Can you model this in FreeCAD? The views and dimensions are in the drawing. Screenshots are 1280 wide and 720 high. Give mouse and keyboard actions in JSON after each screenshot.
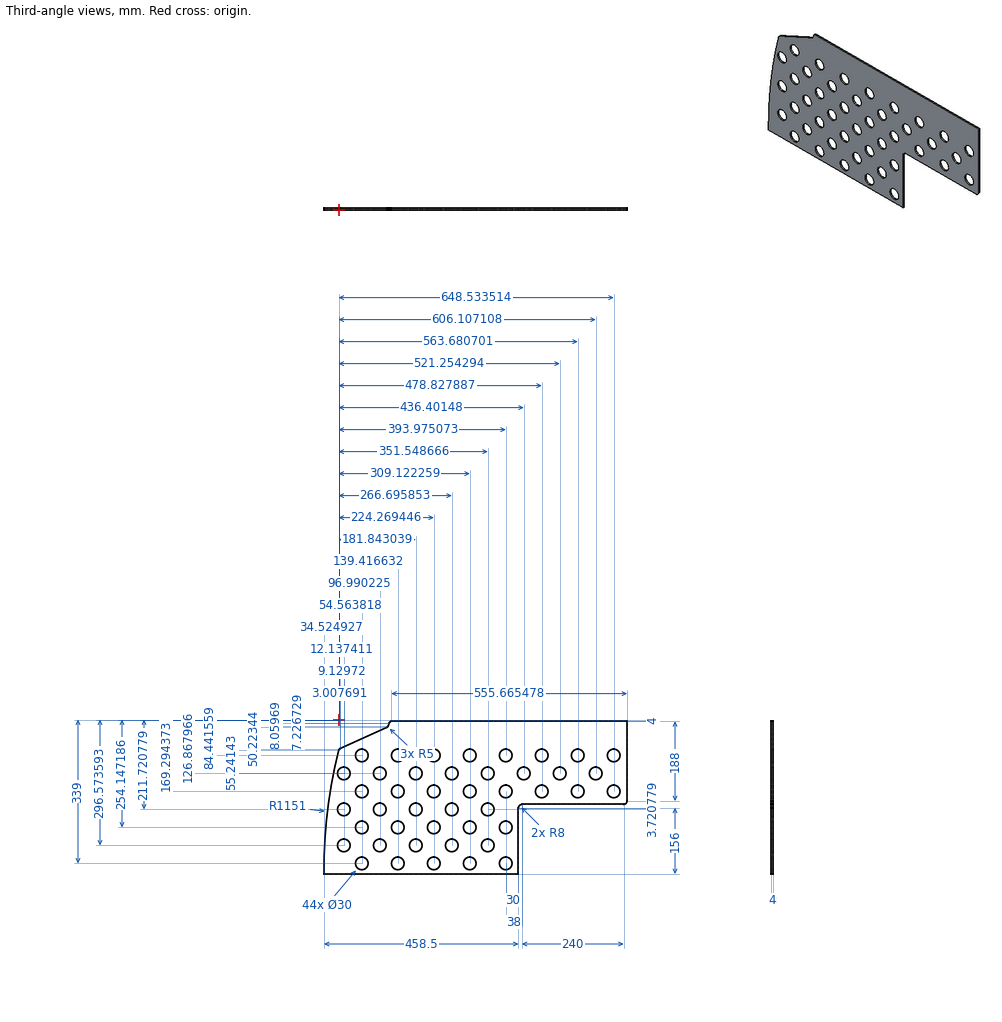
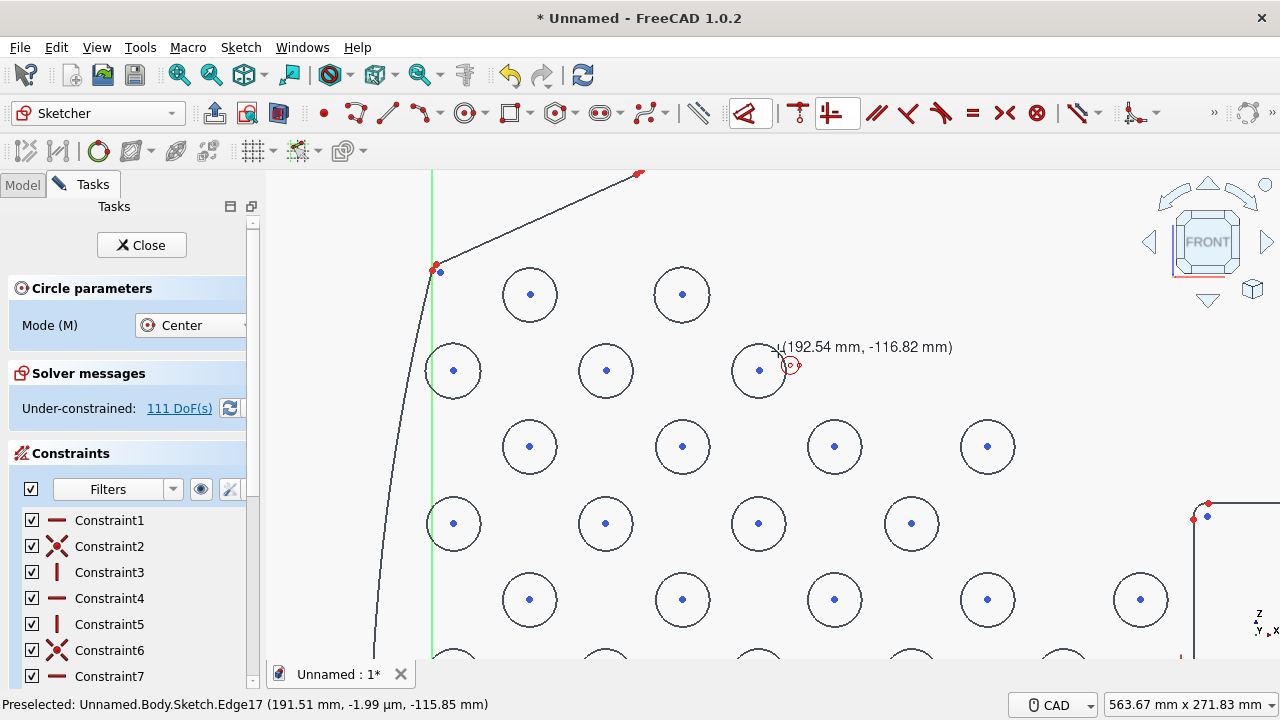
{"action": "left_click", "coordinate": [911, 370]}
{"action": "left_click", "coordinate": [930, 351]}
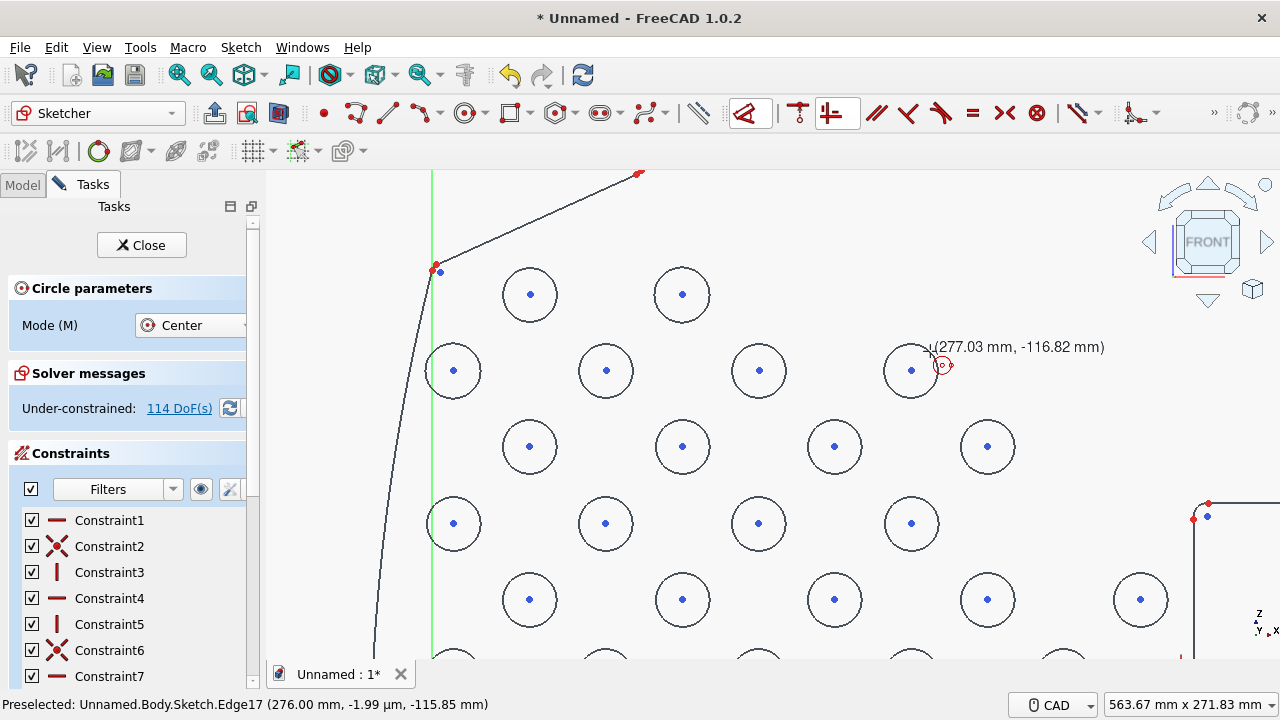
{"action": "left_click", "coordinate": [835, 294]}
{"action": "left_click", "coordinate": [854, 275]}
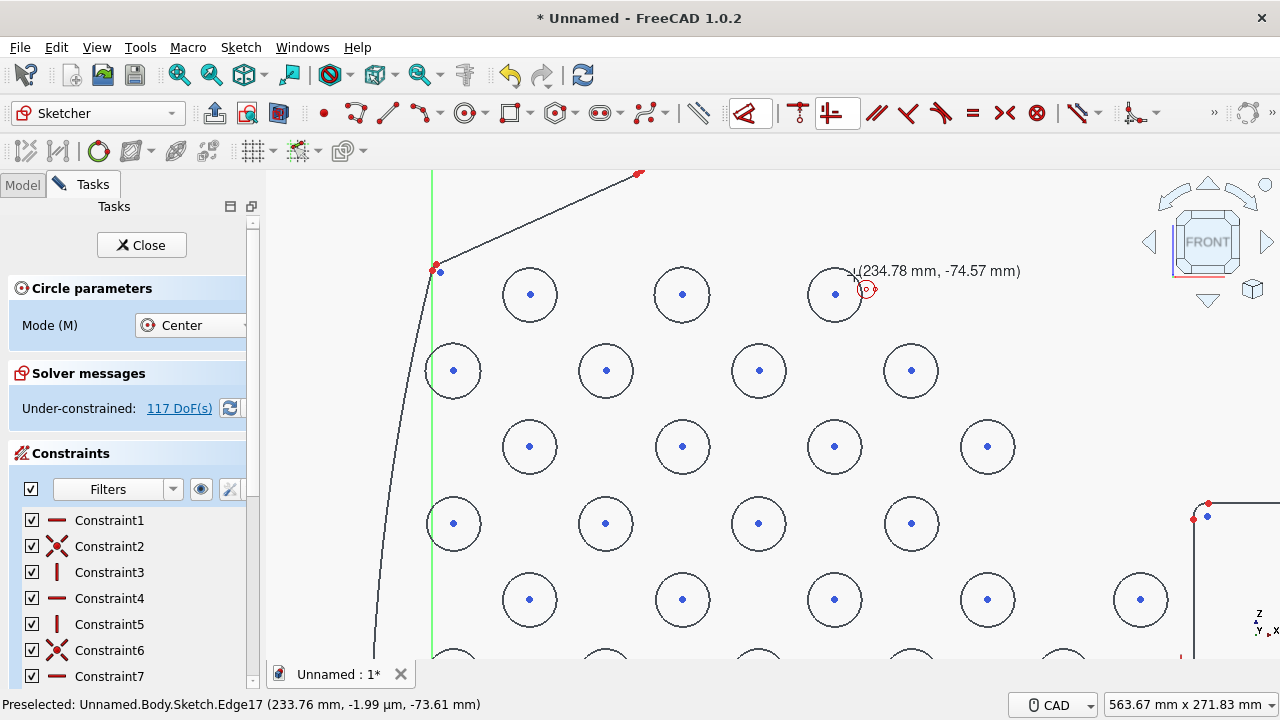
{"action": "left_click", "coordinate": [988, 294]}
{"action": "left_click", "coordinate": [1007, 275]}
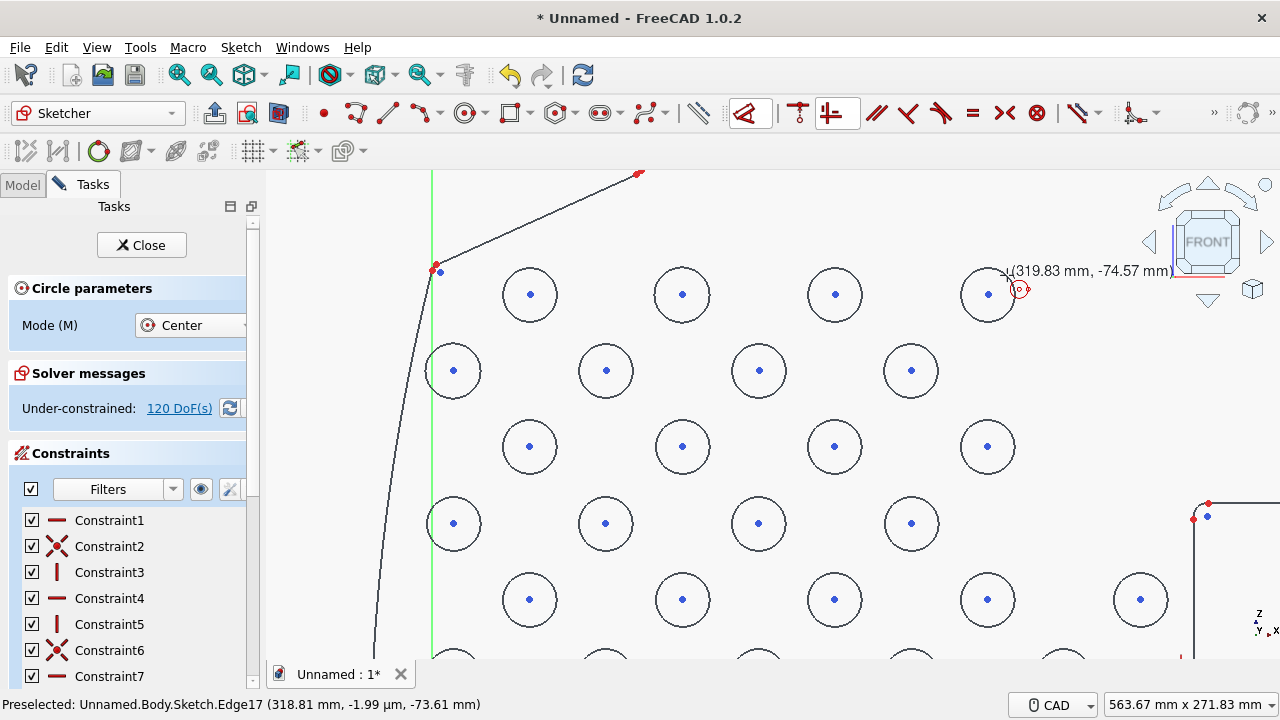
{"action": "left_click", "coordinate": [1064, 523]}
{"action": "left_click", "coordinate": [1083, 504]}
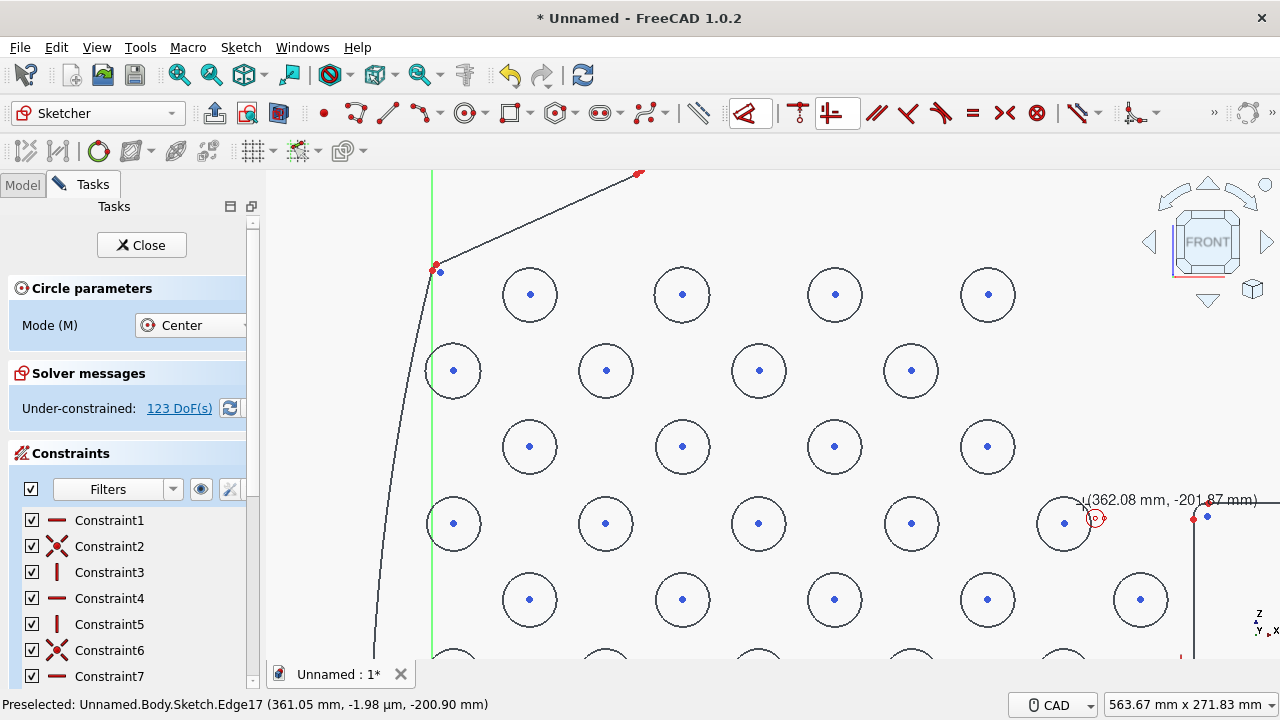
{"action": "scroll", "coordinate": [453, 370], "scroll_direction": "down", "scroll_amount": 4}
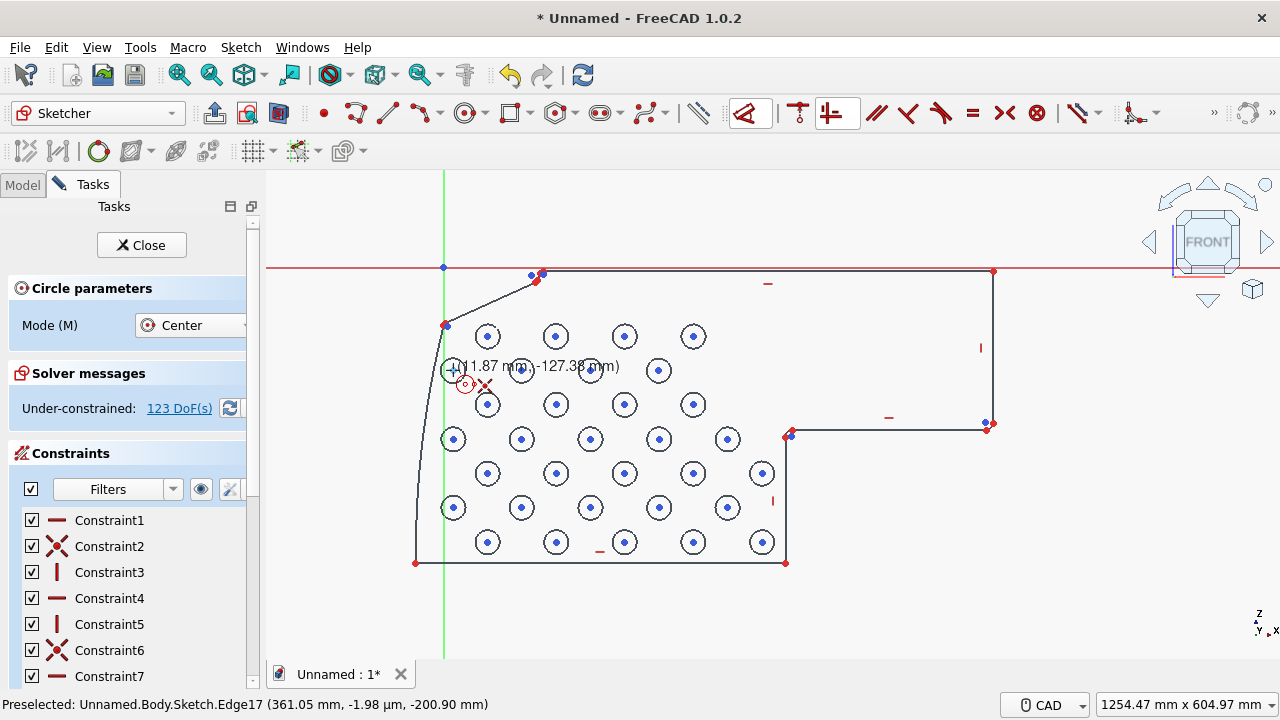
{"action": "scroll", "coordinate": [762, 405], "scroll_direction": "up", "scroll_amount": 4}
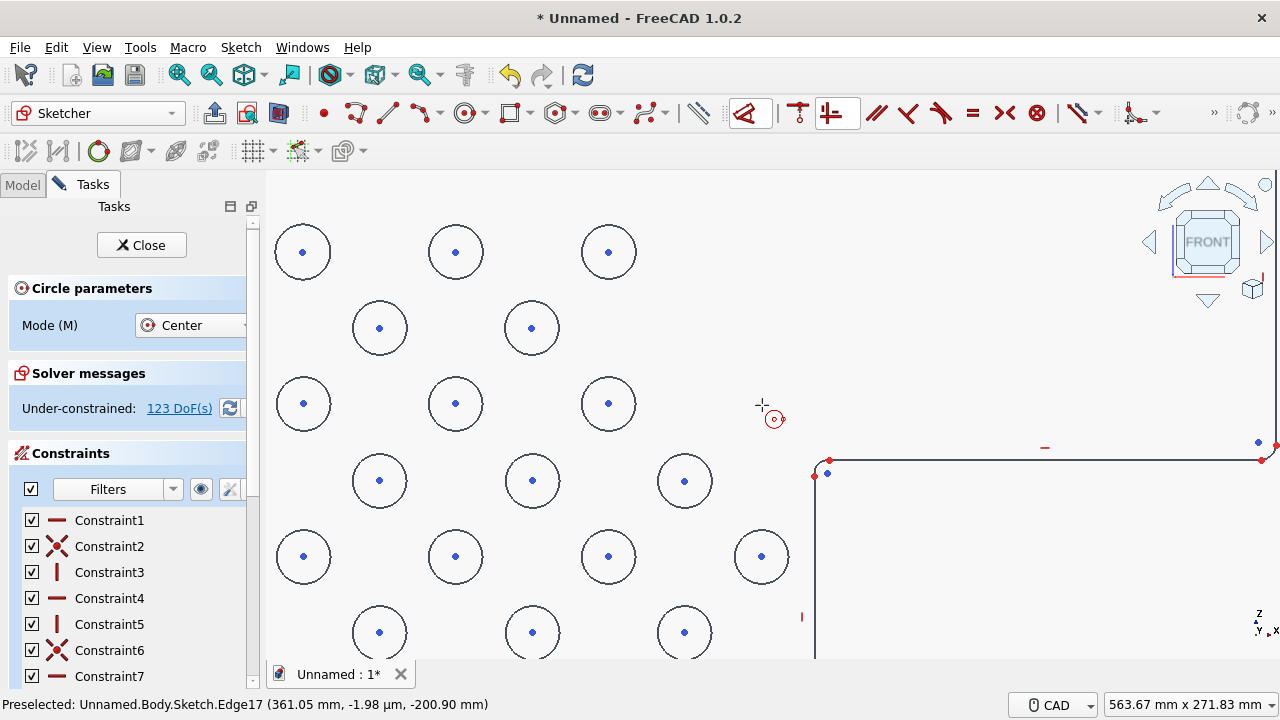
{"action": "left_click", "coordinate": [761, 403]}
{"action": "left_click", "coordinate": [780, 384]}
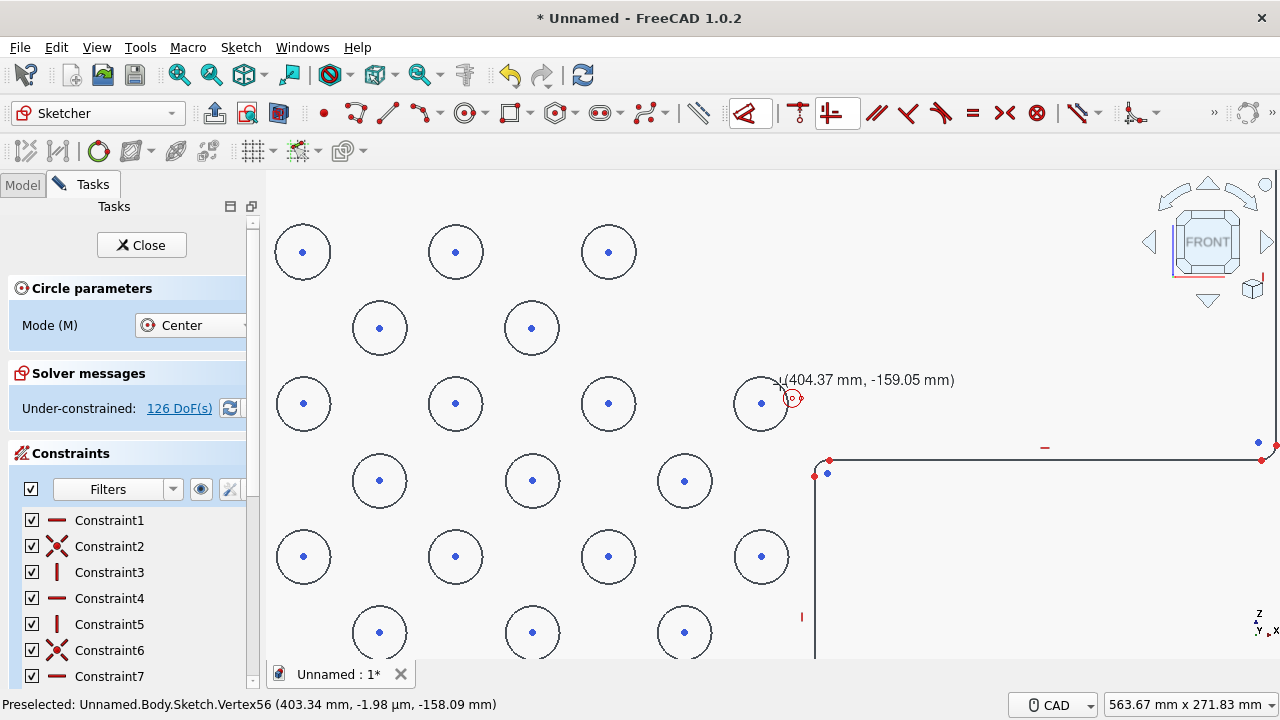
{"action": "left_click", "coordinate": [914, 403]}
{"action": "left_click", "coordinate": [933, 384]}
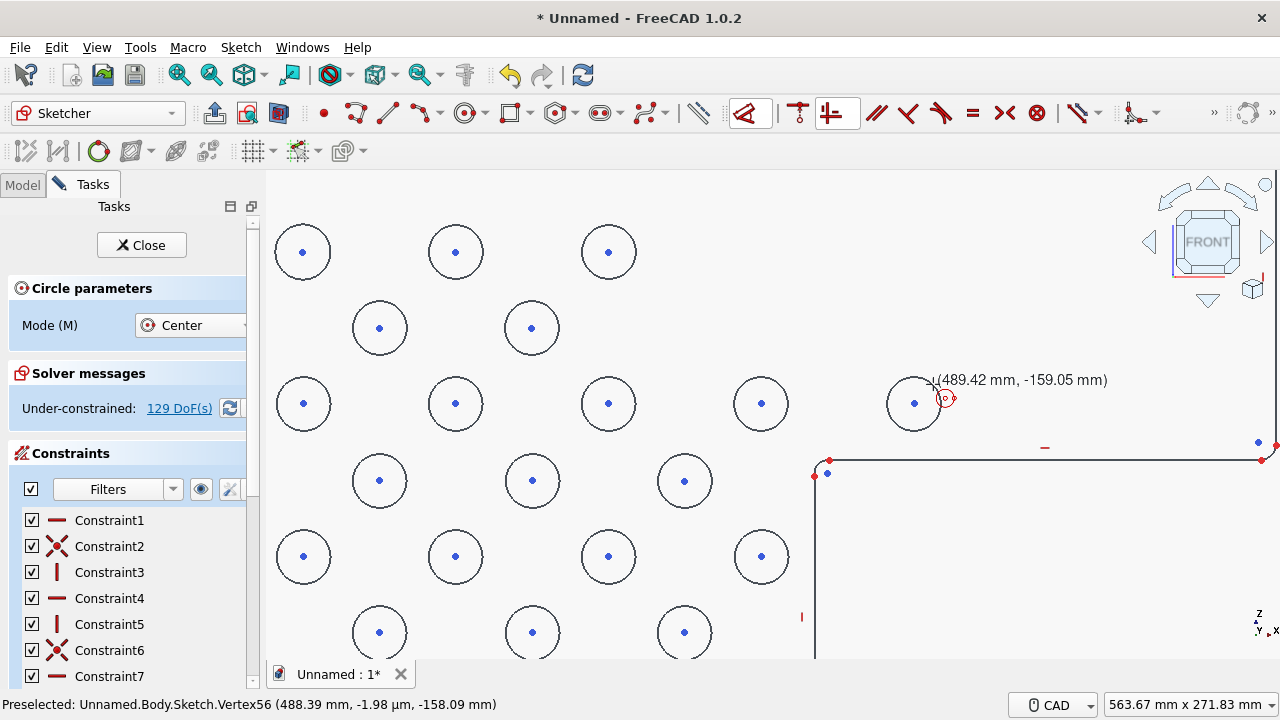
{"action": "left_click", "coordinate": [1067, 403]}
{"action": "left_click", "coordinate": [1086, 384]}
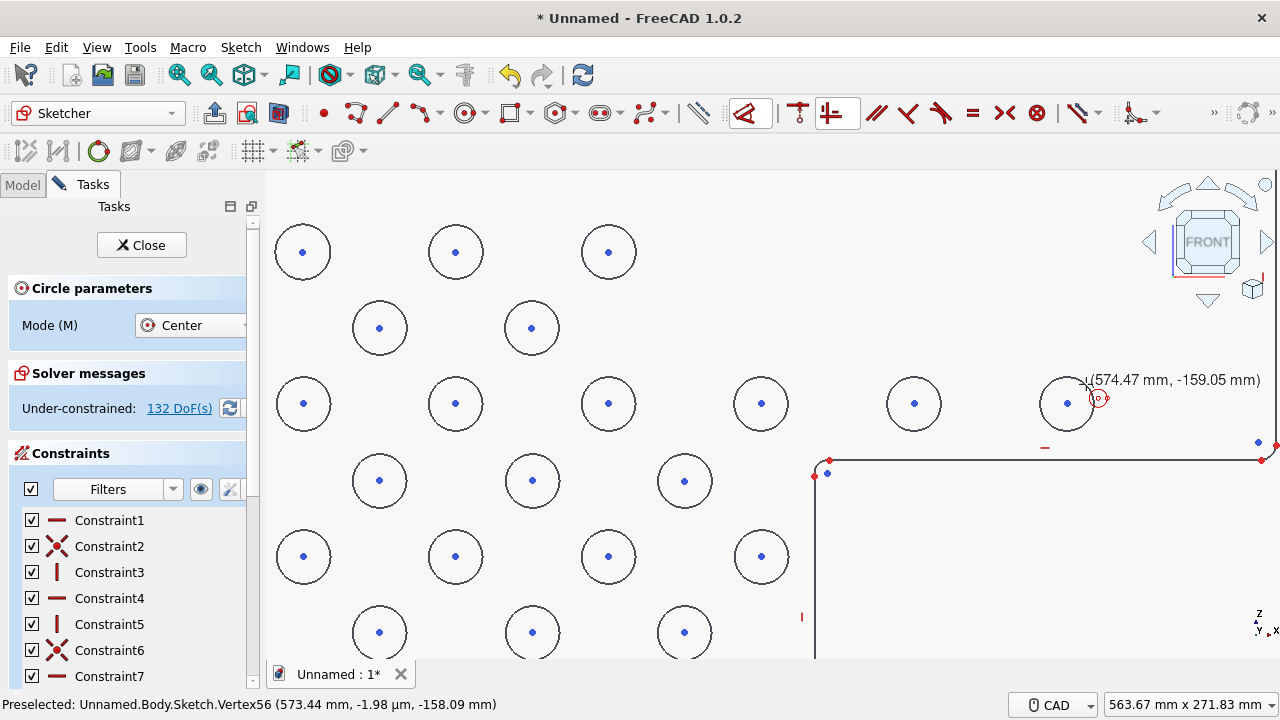
{"action": "scroll", "coordinate": [763, 405], "scroll_direction": "down", "scroll_amount": 4}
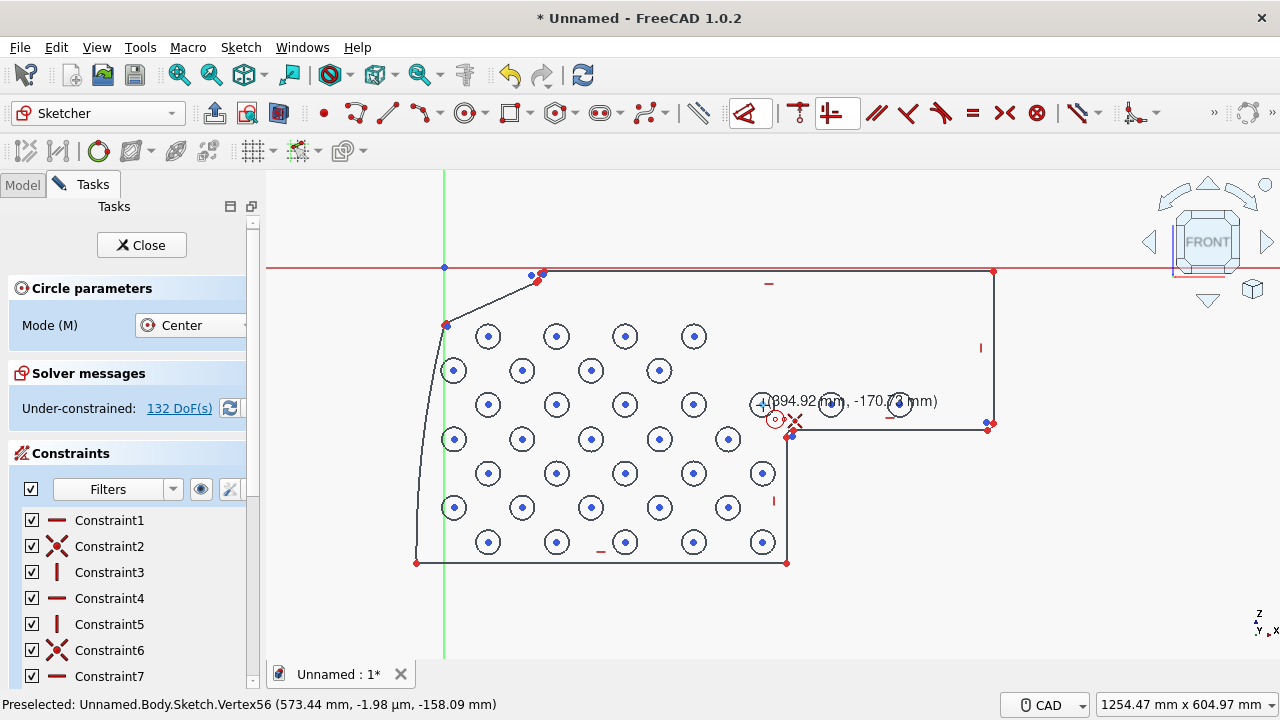
{"action": "scroll", "coordinate": [968, 405], "scroll_direction": "up", "scroll_amount": 4}